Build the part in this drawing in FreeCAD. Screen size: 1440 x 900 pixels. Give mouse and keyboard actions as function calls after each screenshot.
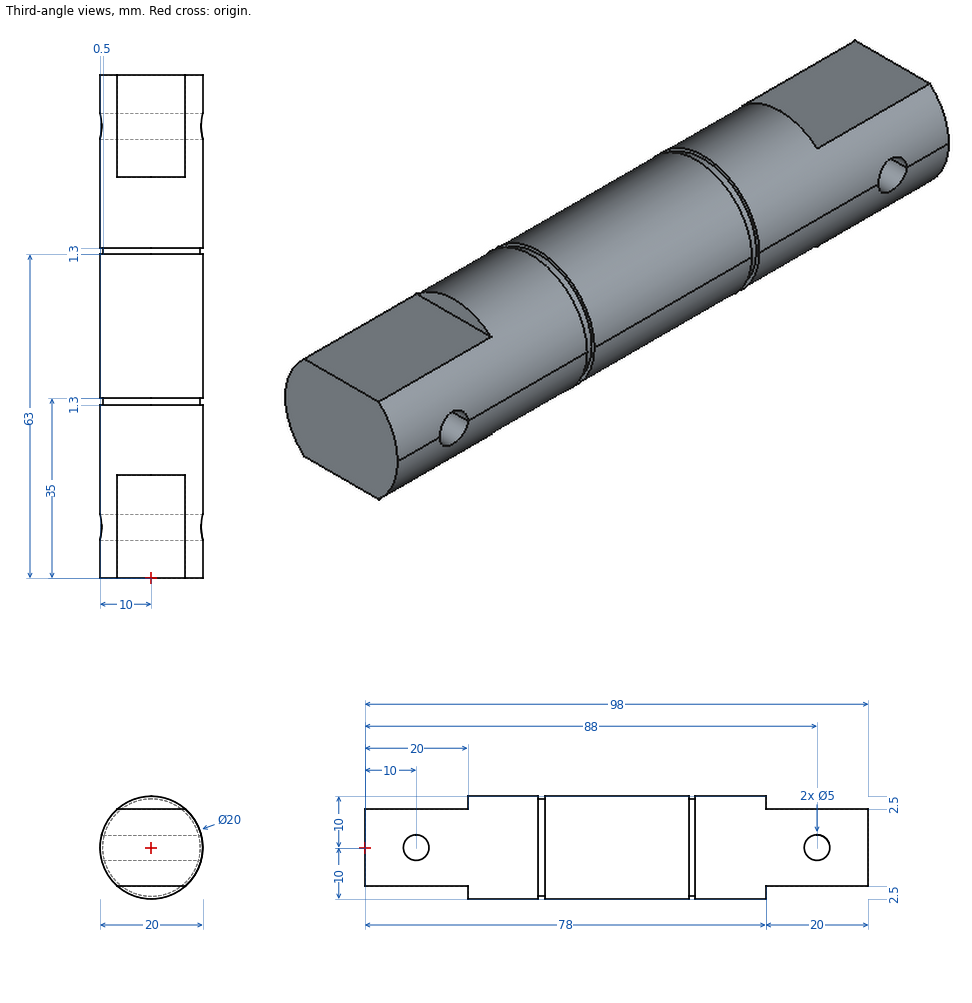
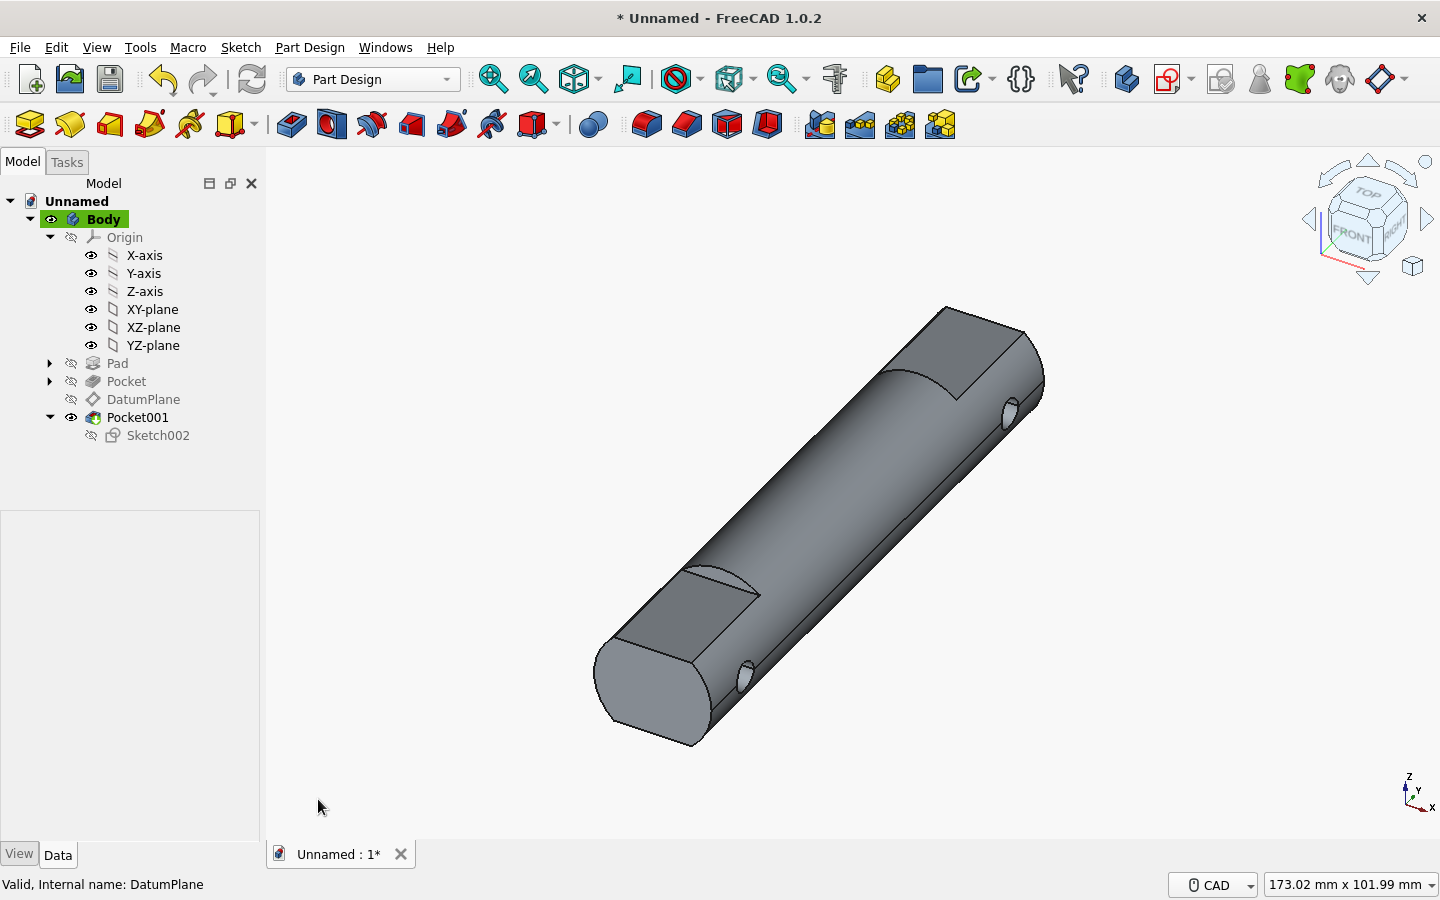
click(1168, 80)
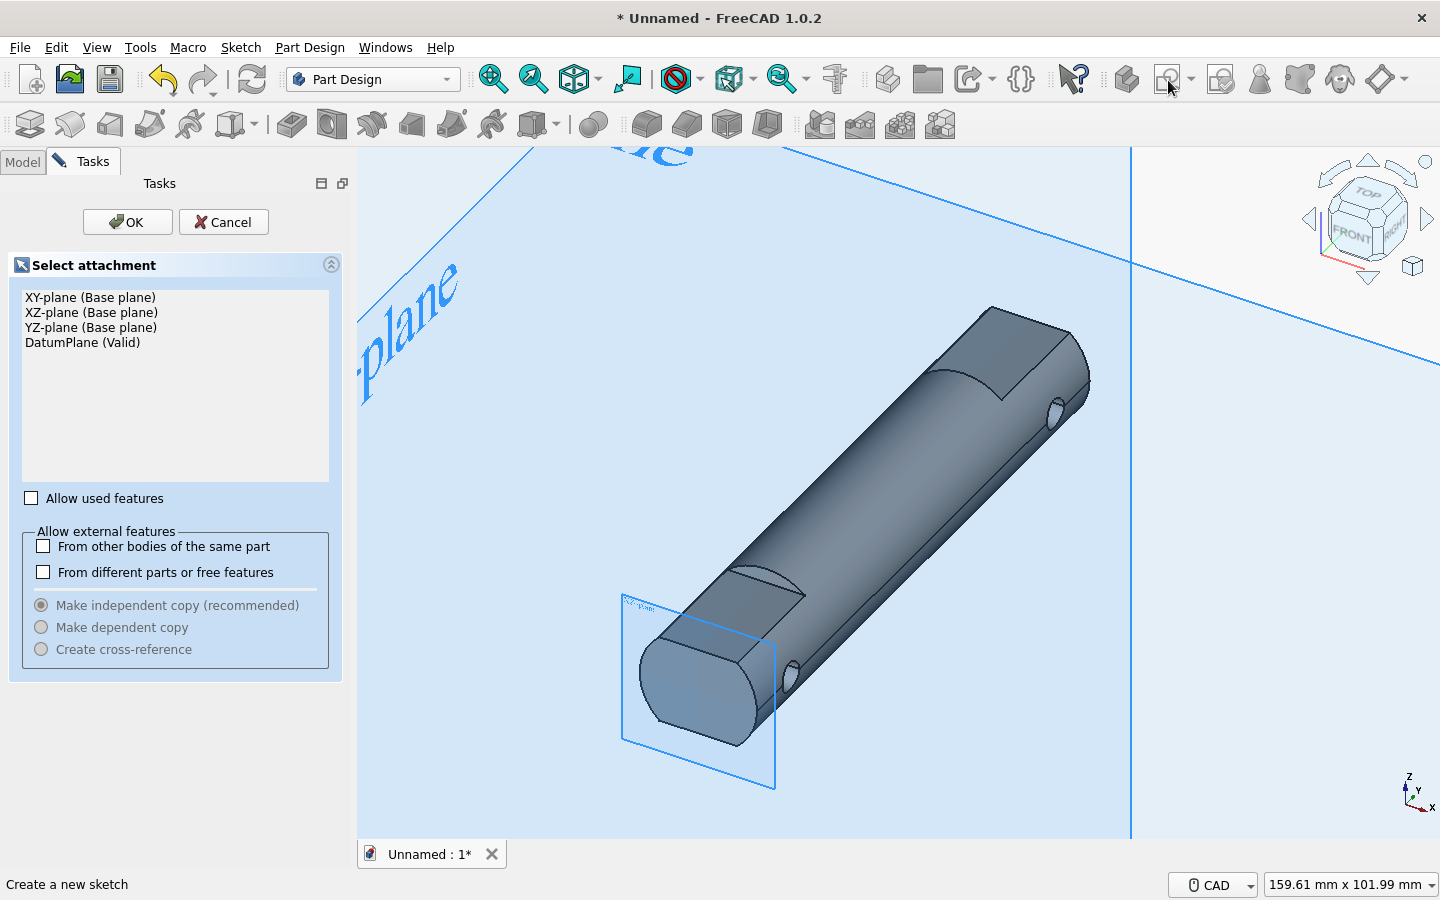
click(82, 298)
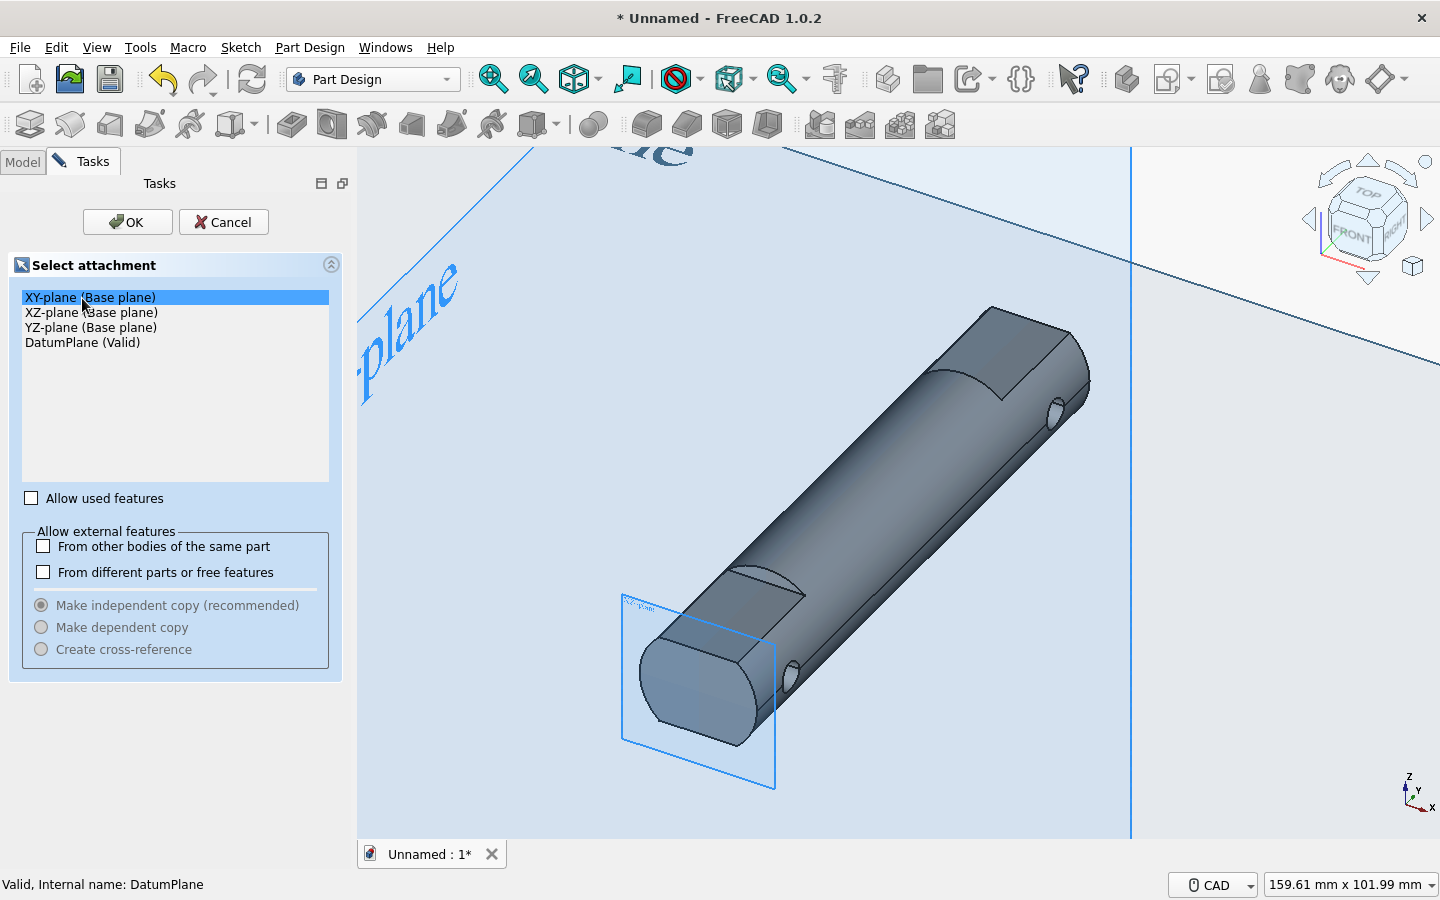
click(128, 222)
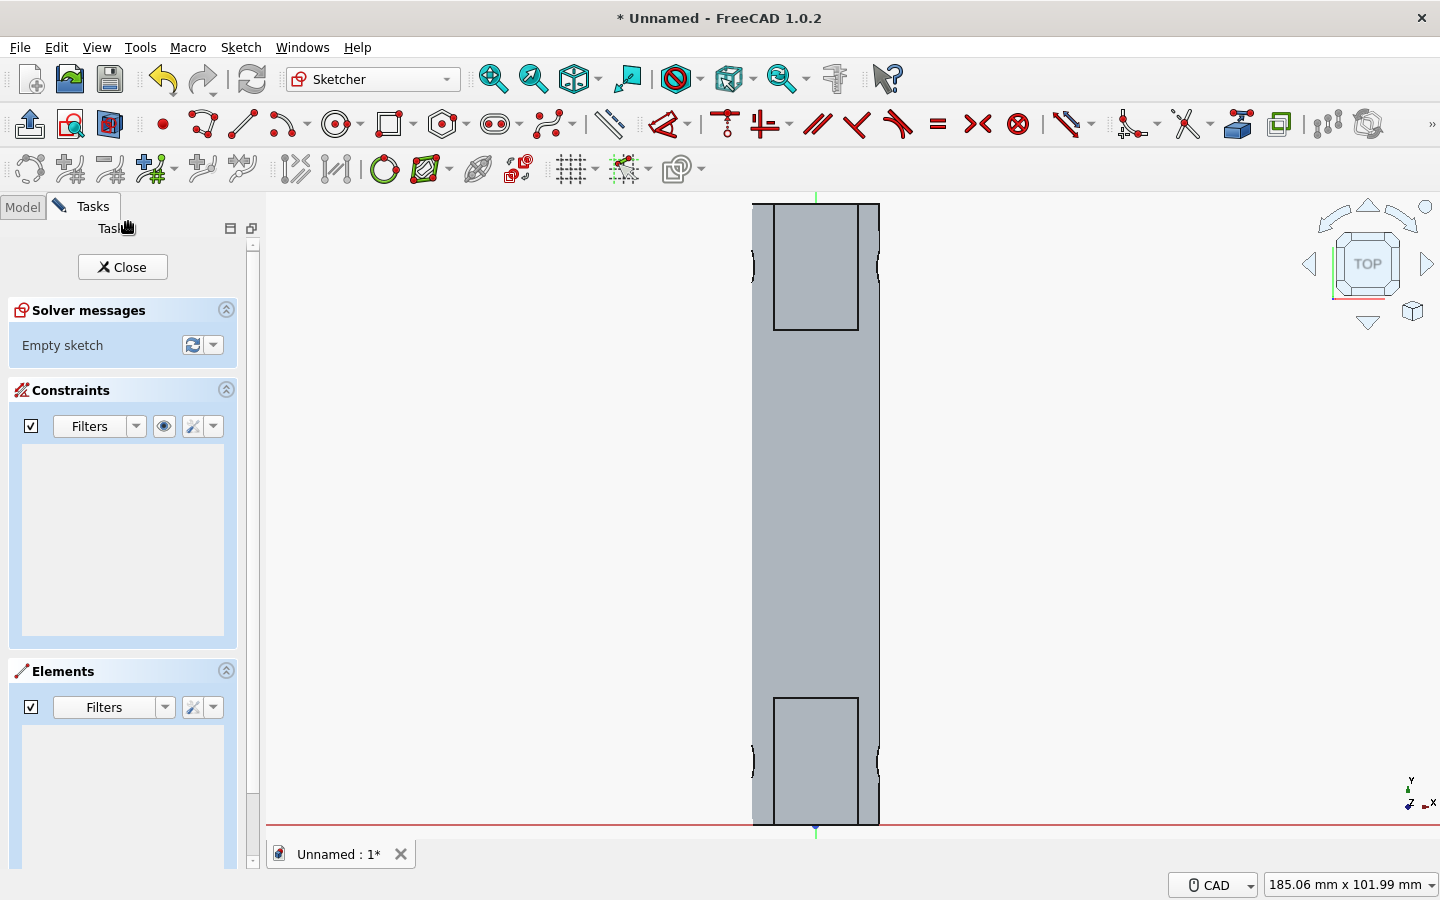
click(110, 124)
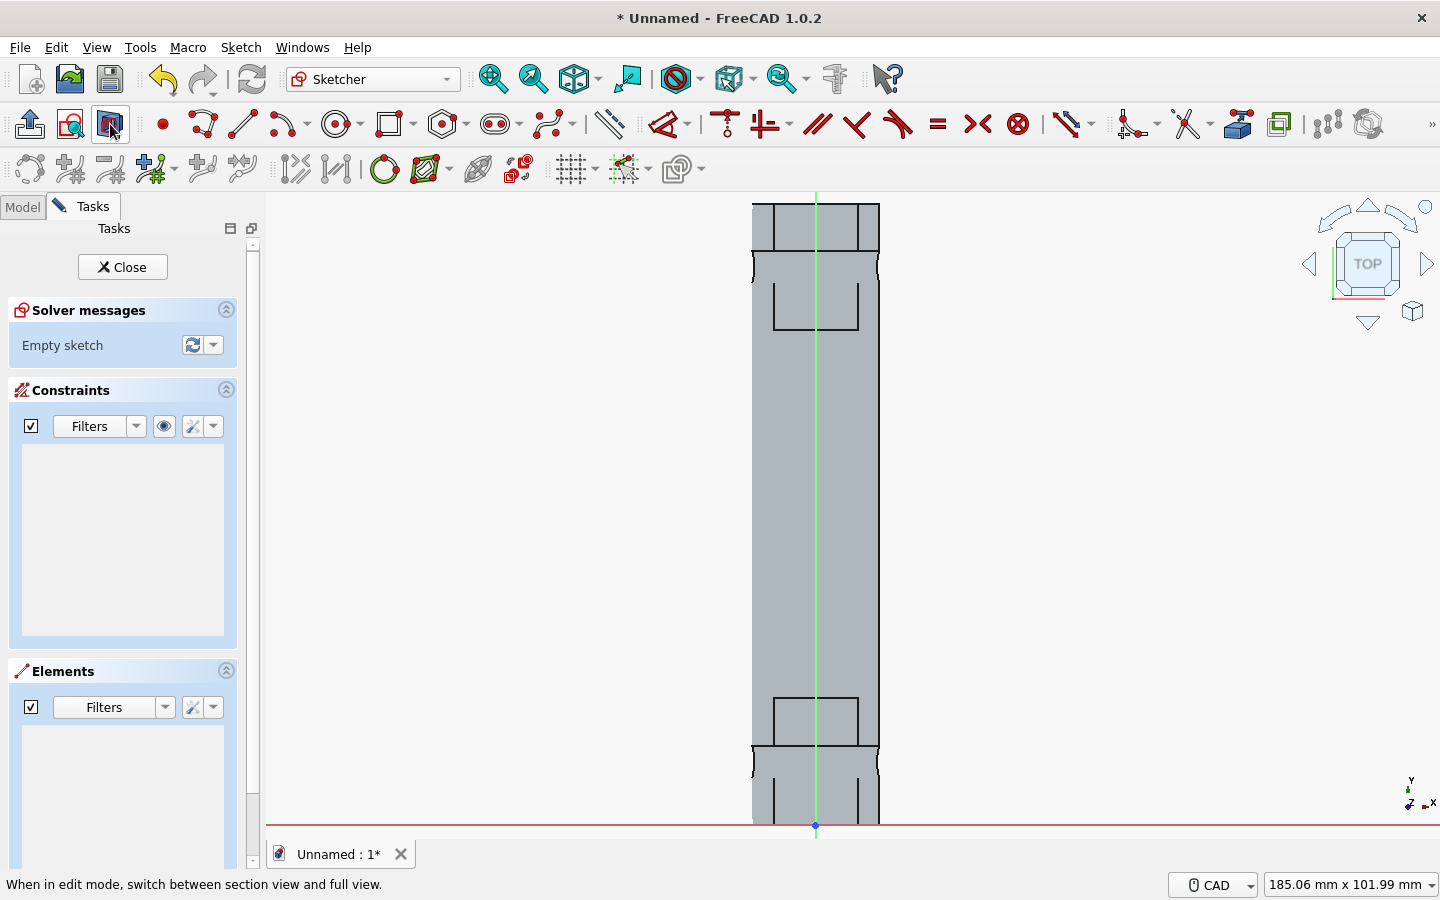
scroll(787, 220, down, 1)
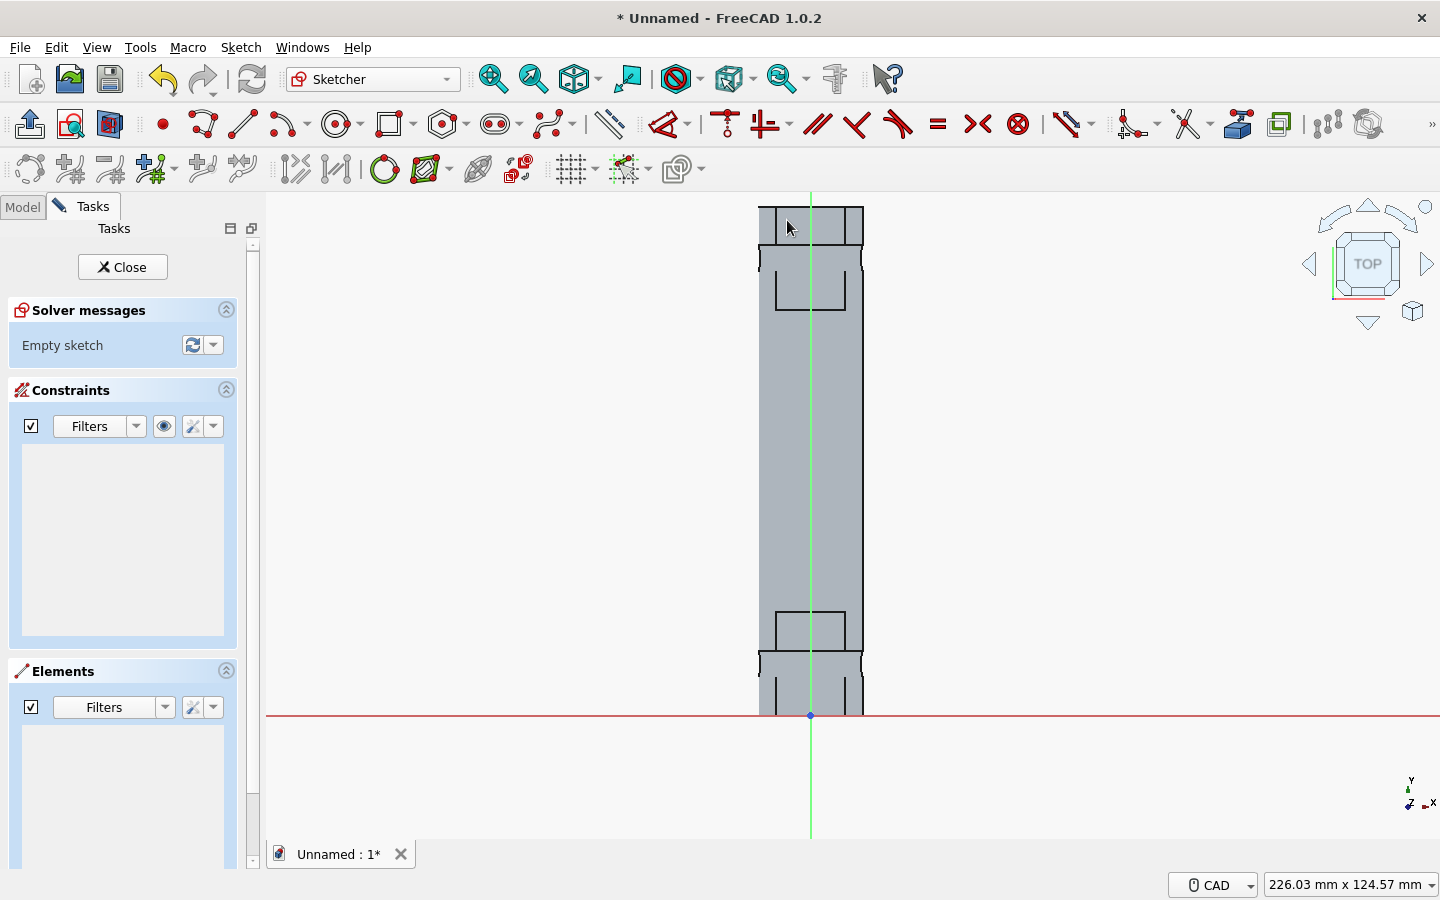
key(g)
key(r)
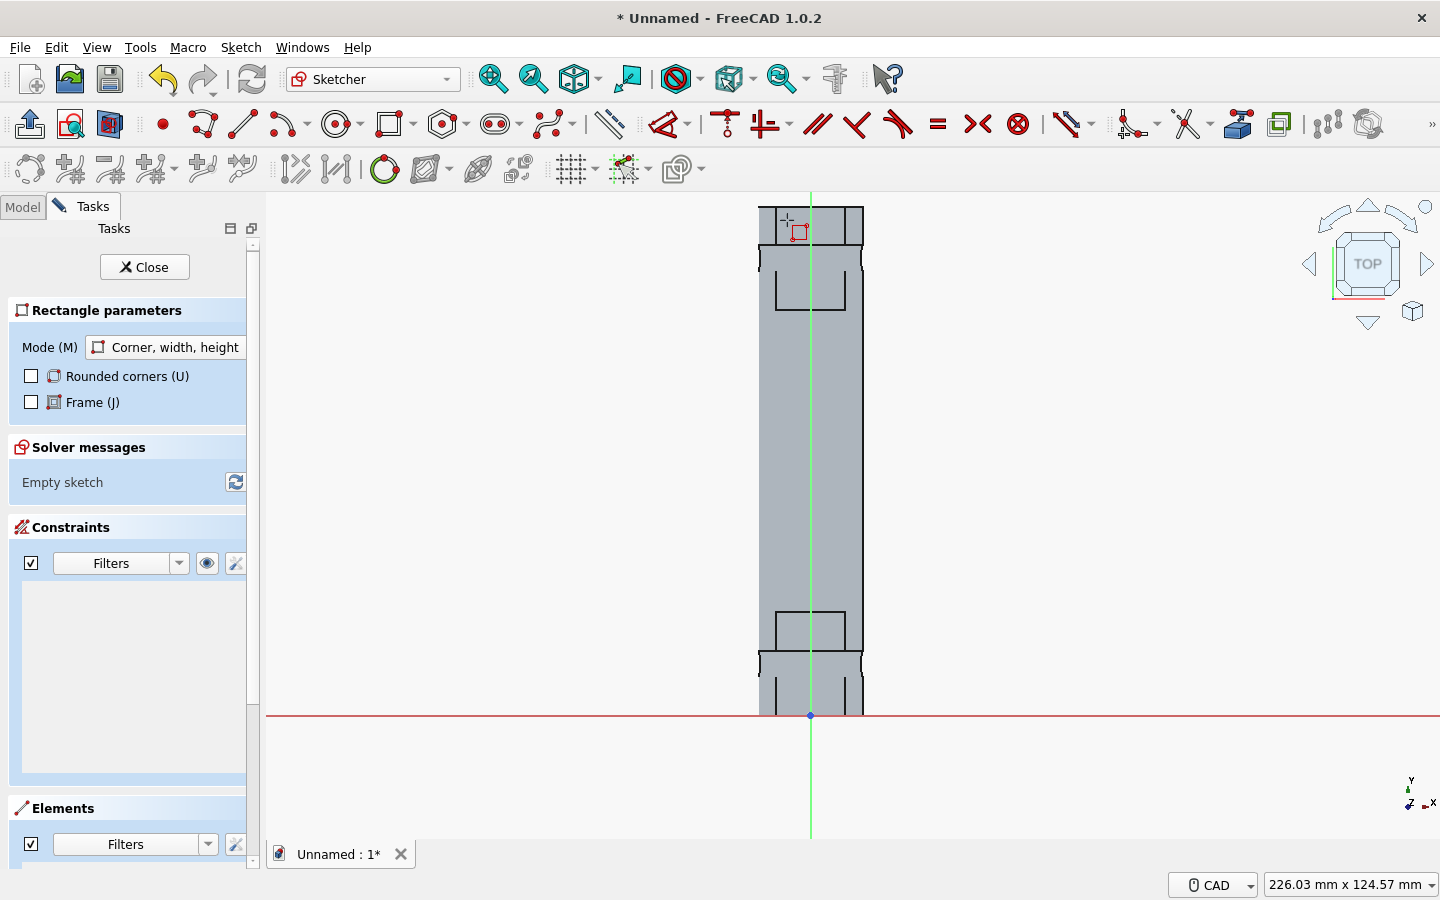
scroll(759, 382, up, 10)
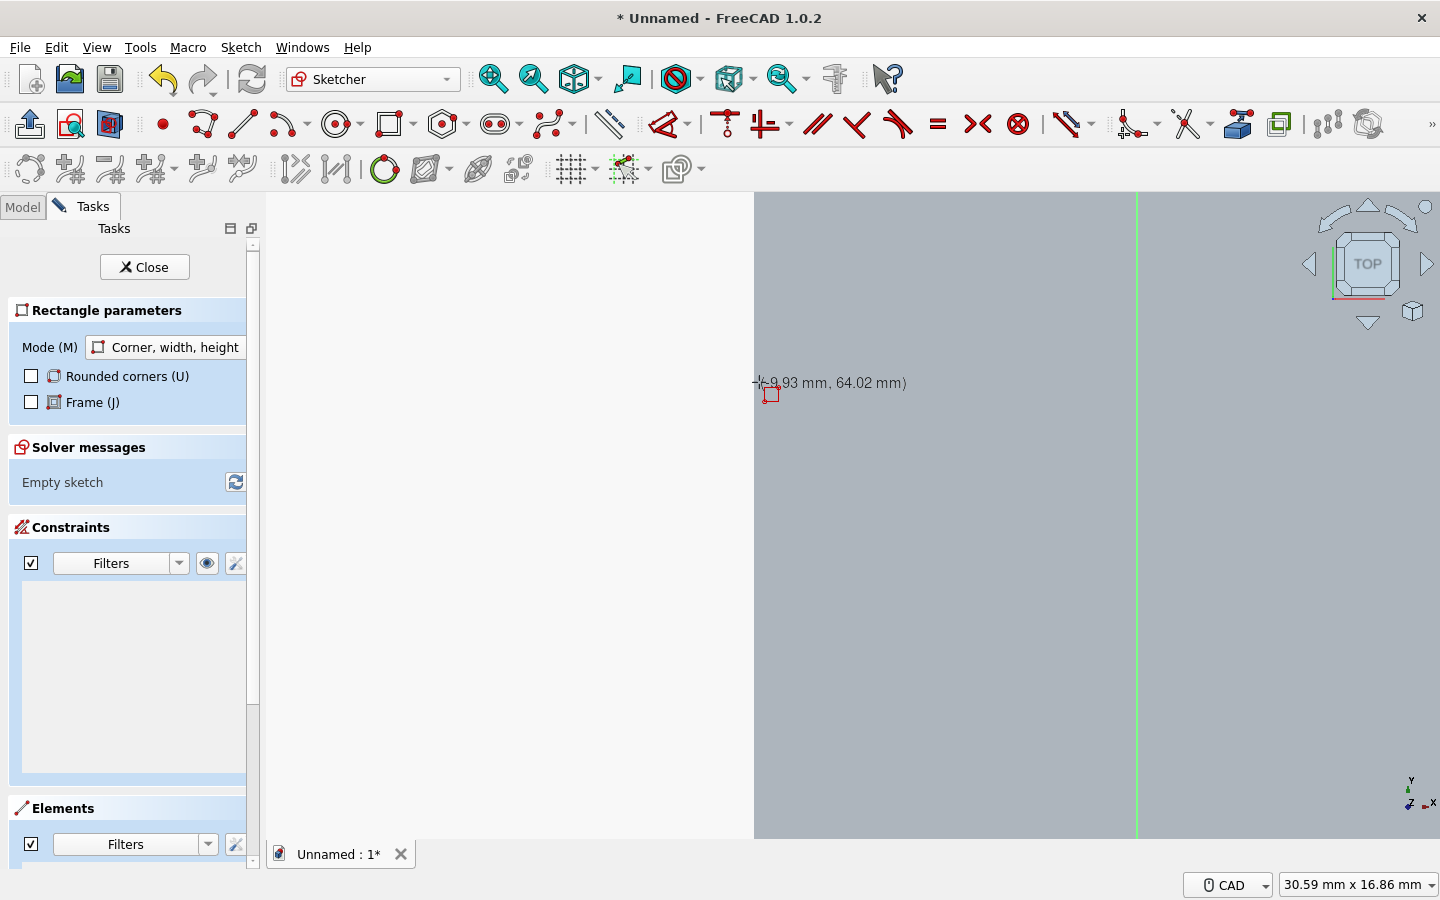
scroll(753, 299, down, 9)